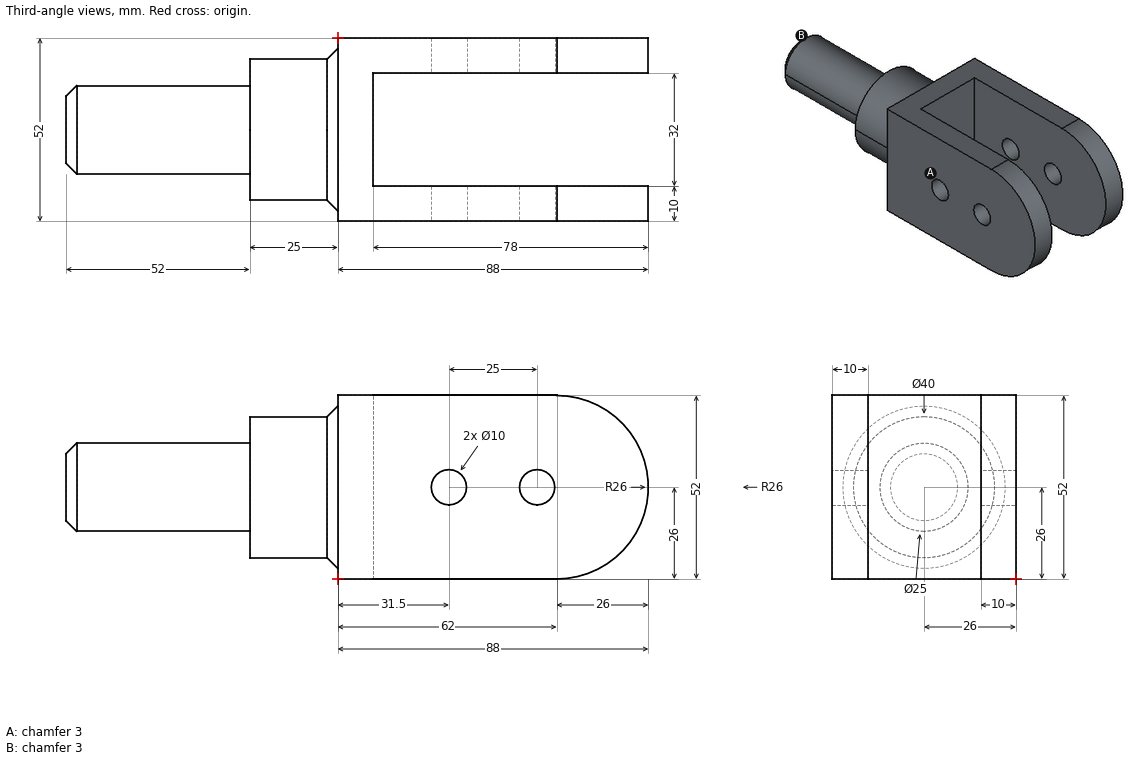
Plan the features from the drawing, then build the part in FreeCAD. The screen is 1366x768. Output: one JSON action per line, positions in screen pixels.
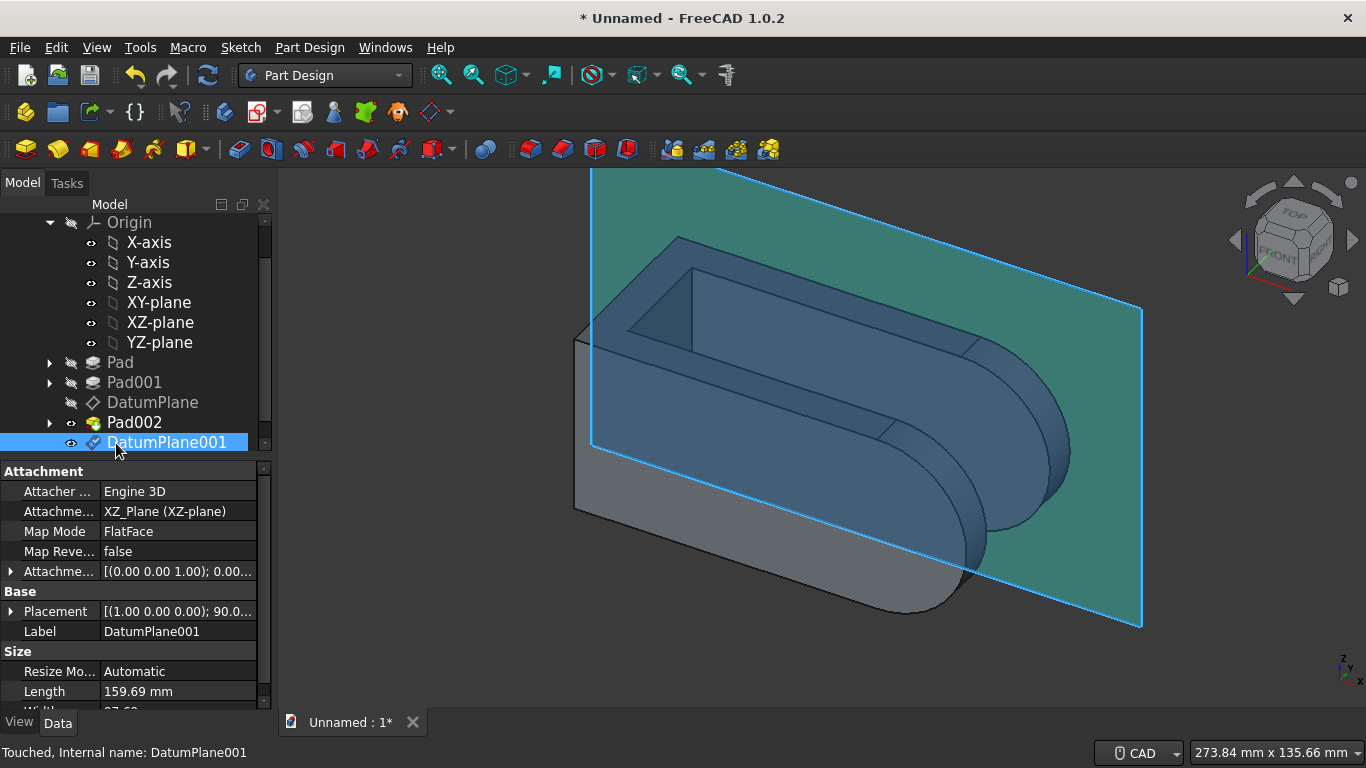
{"action": "left_click", "coordinate": [258, 112]}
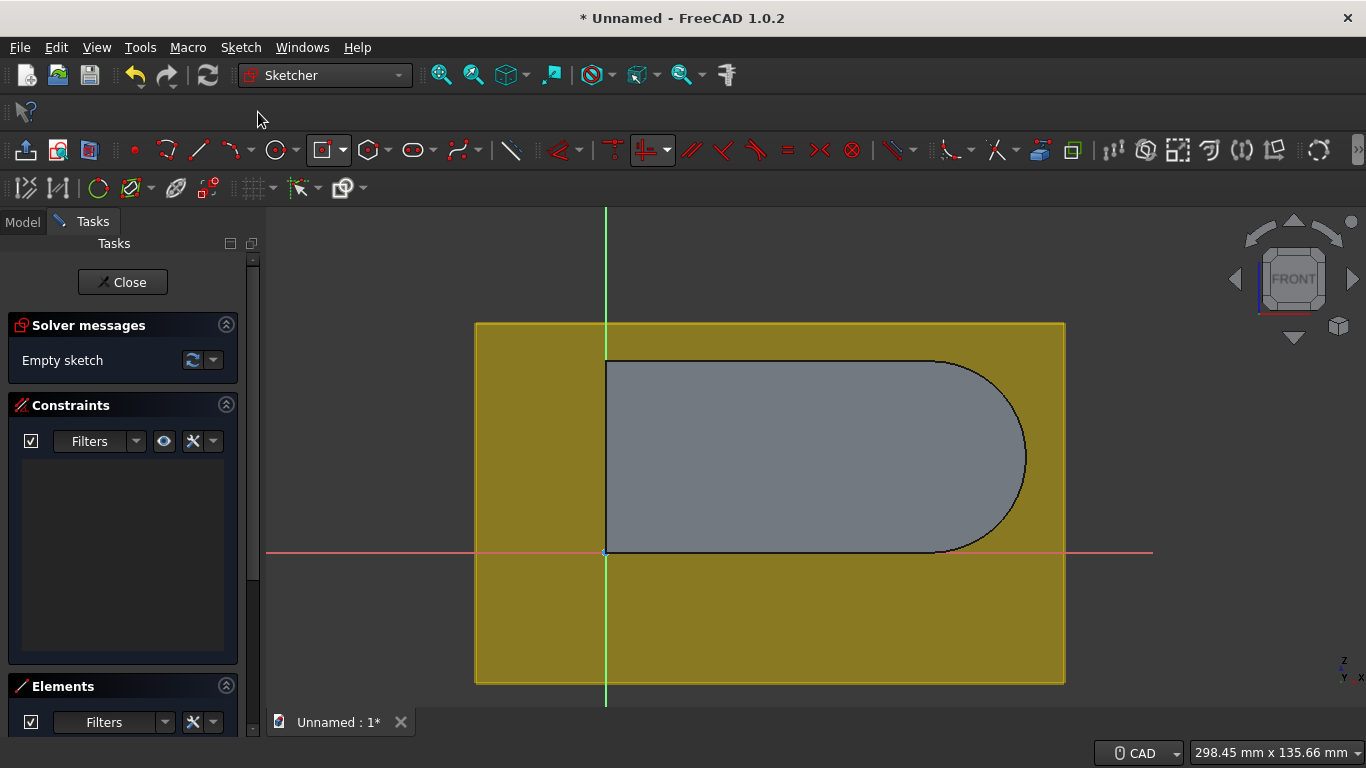
{"action": "left_click", "coordinate": [90, 150]}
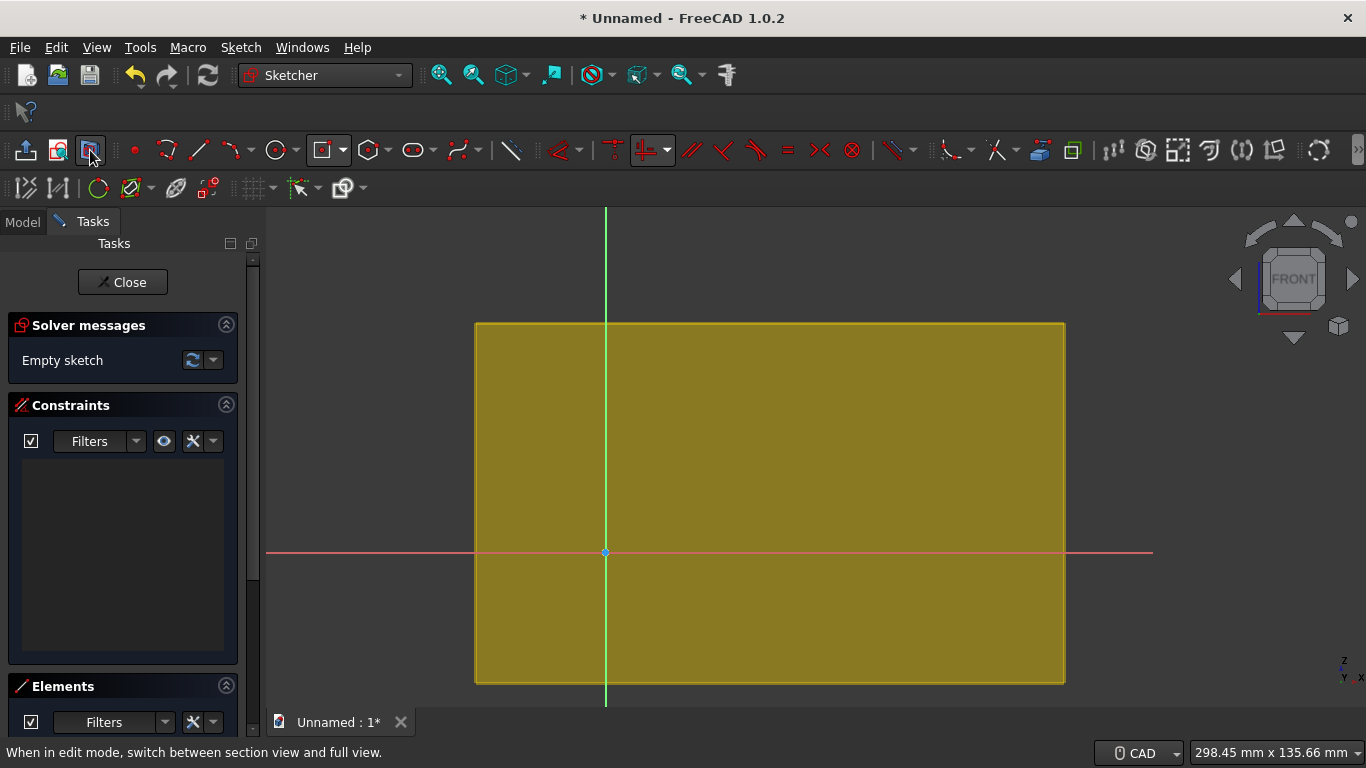
{"action": "scroll", "coordinate": [955, 457], "scroll_direction": "up", "scroll_amount": 2}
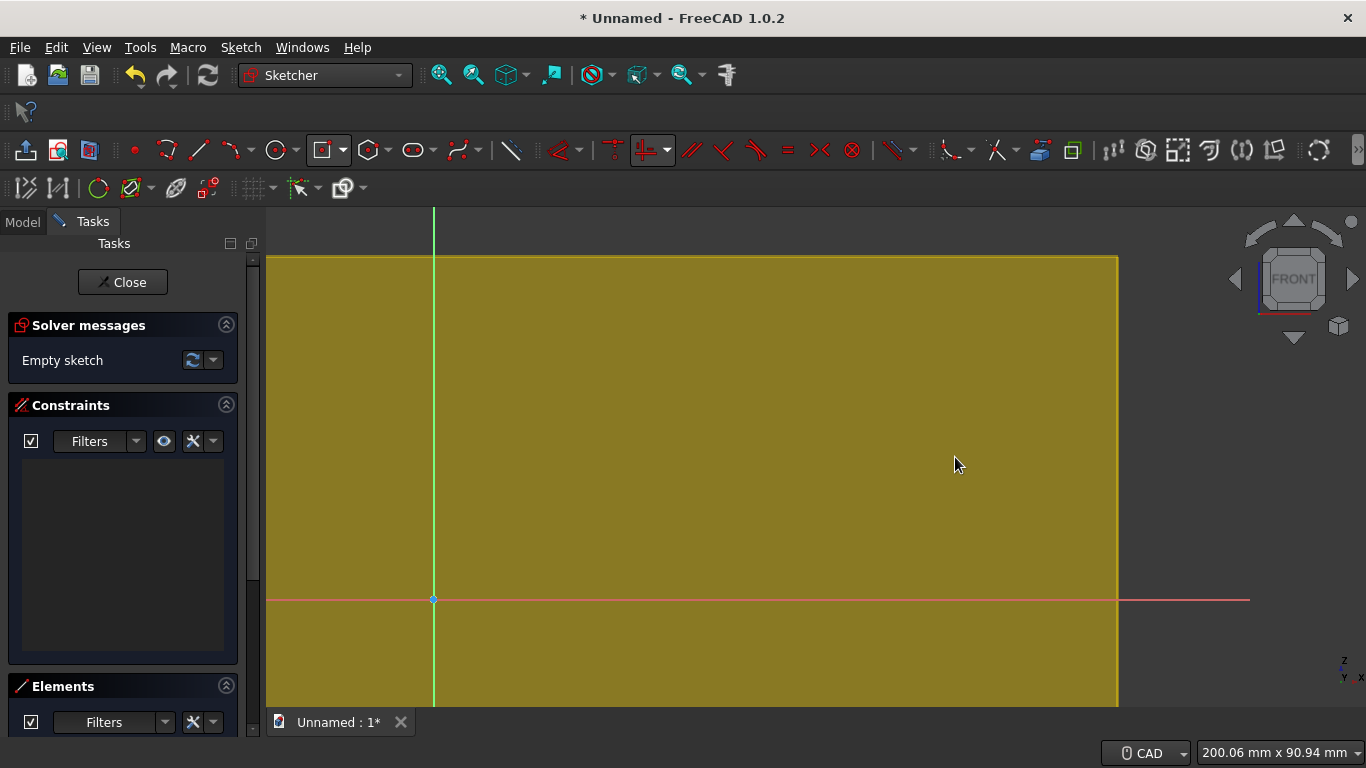
{"action": "left_click", "coordinate": [200, 150]}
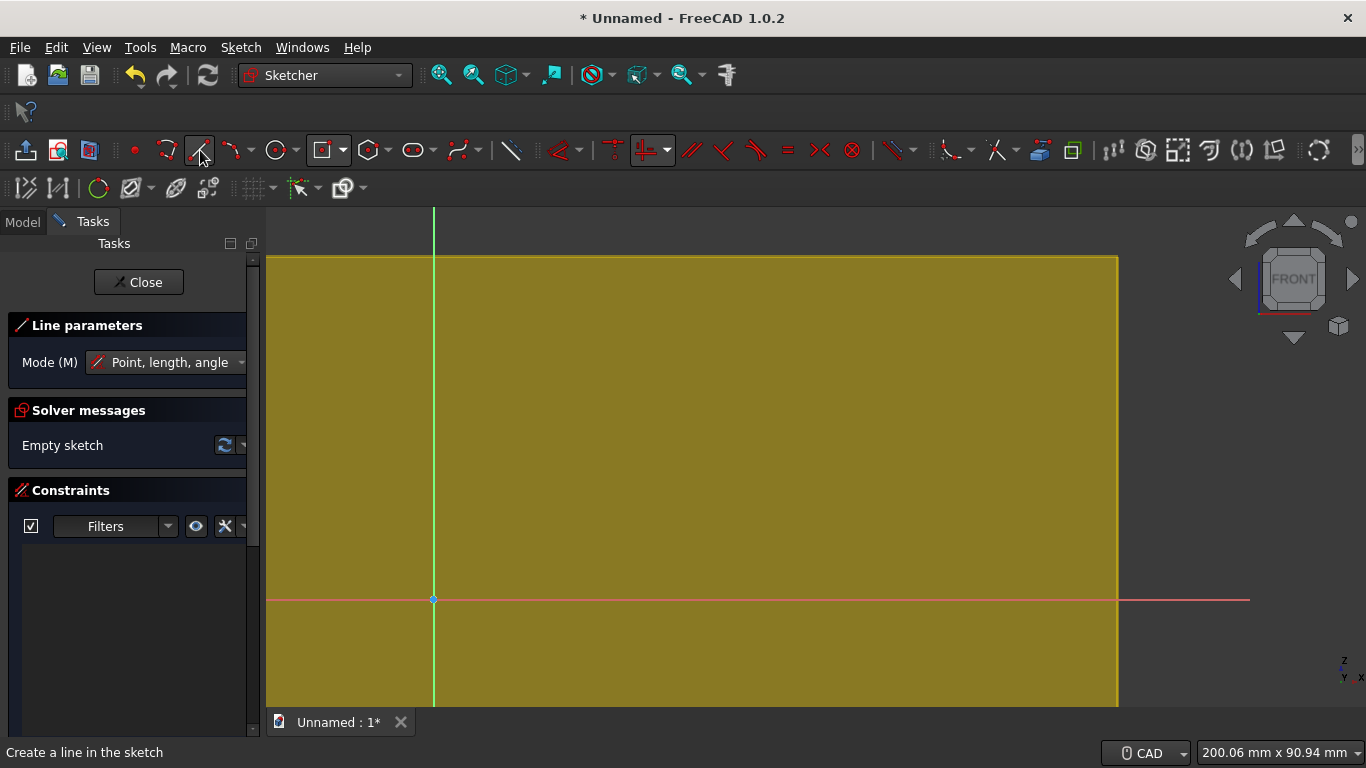
{"action": "left_click", "coordinate": [918, 314]}
{"action": "left_click", "coordinate": [918, 600]}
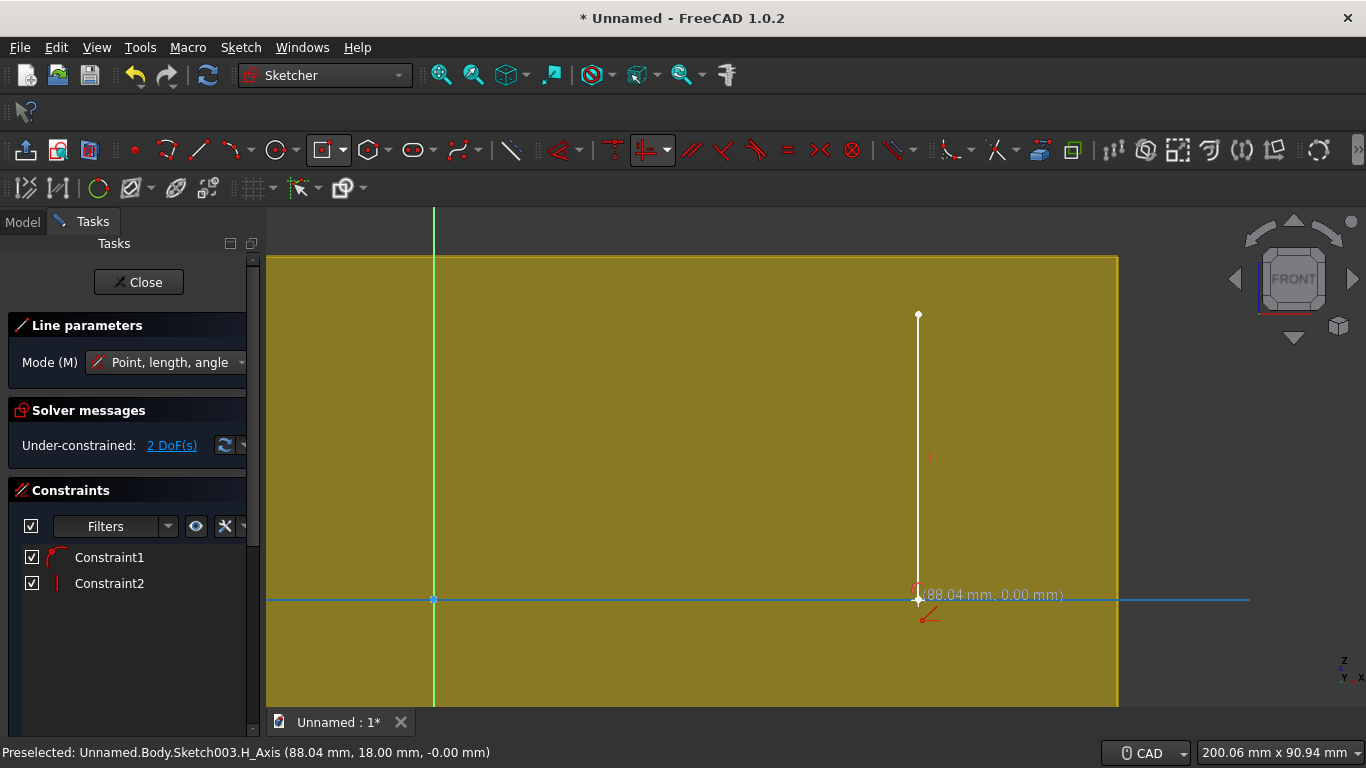
{"action": "left_click", "coordinate": [232, 150]}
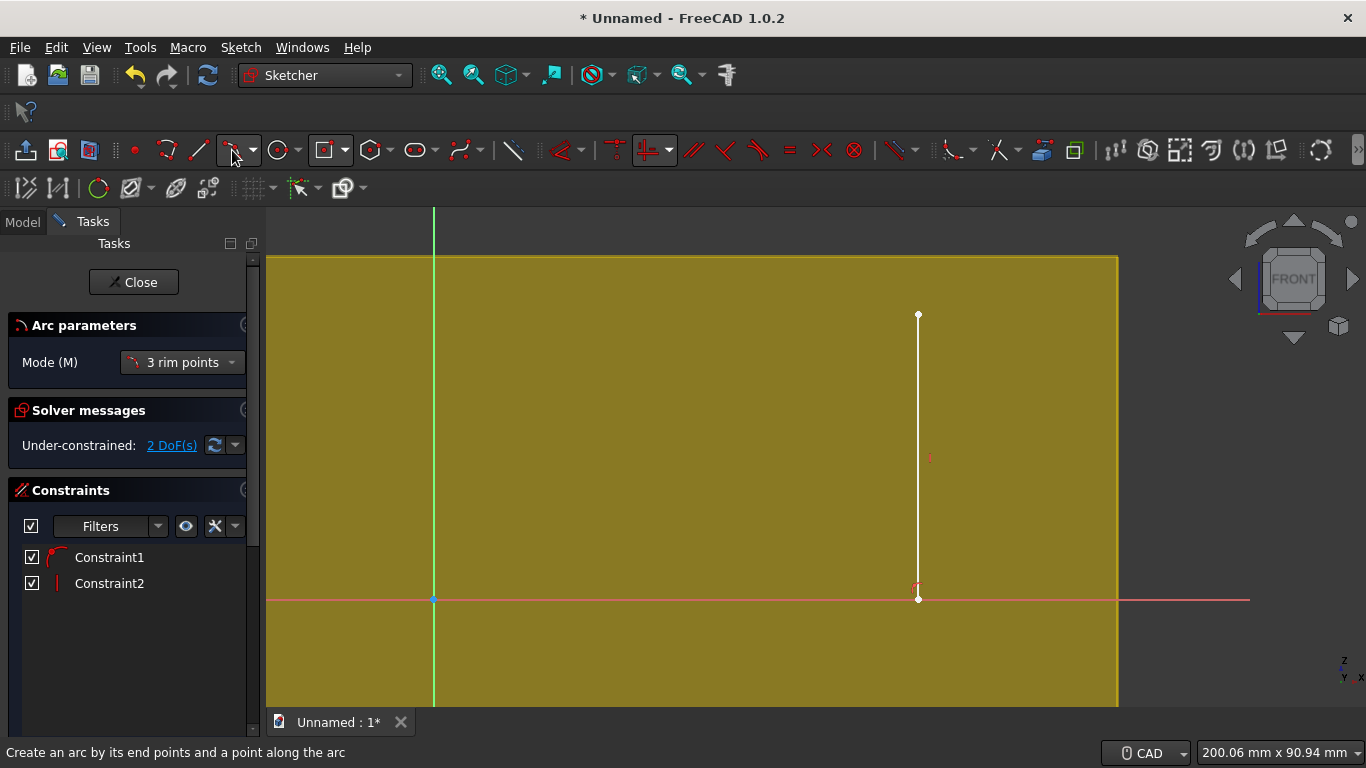
{"action": "left_click", "coordinate": [918, 600]}
{"action": "left_click", "coordinate": [918, 315]}
{"action": "left_click", "coordinate": [1061, 457]}
{"action": "key", "text": "Escape"}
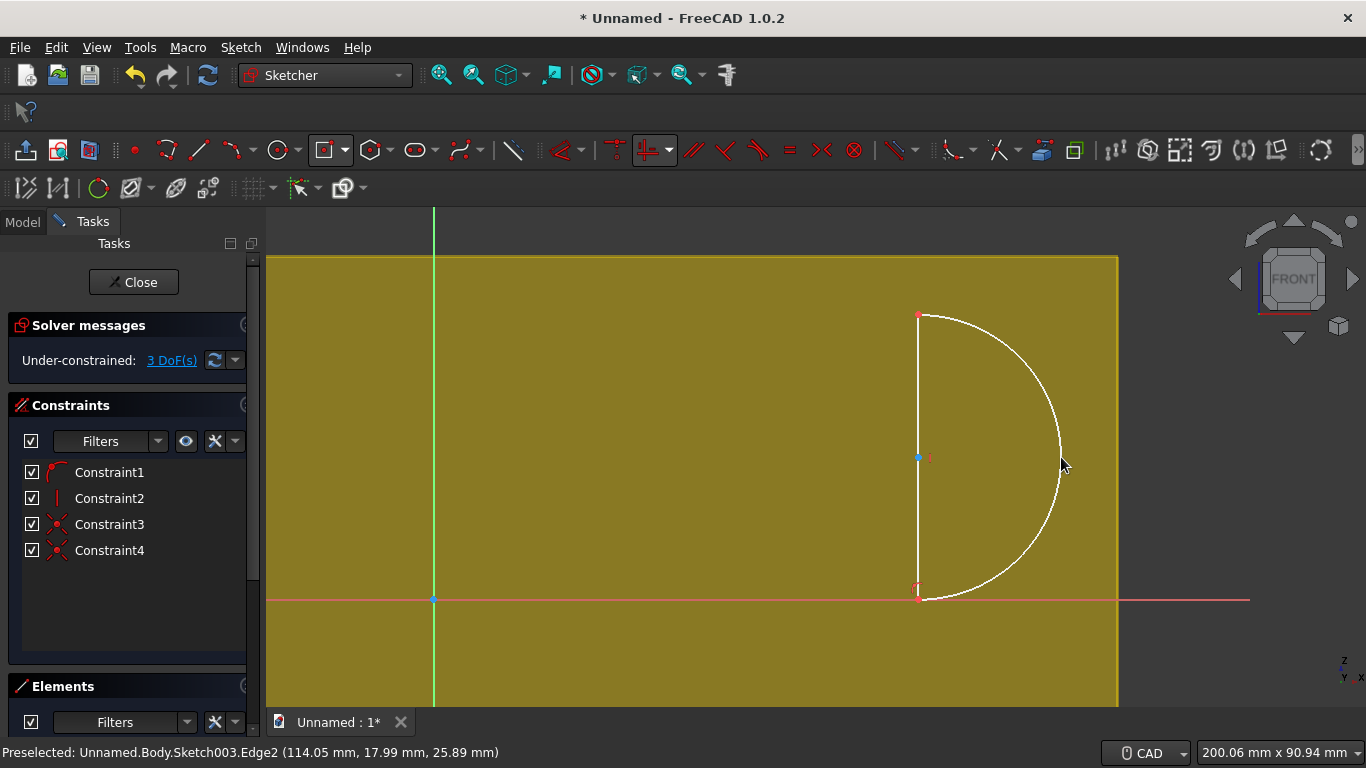
{"action": "left_click", "coordinate": [560, 150]}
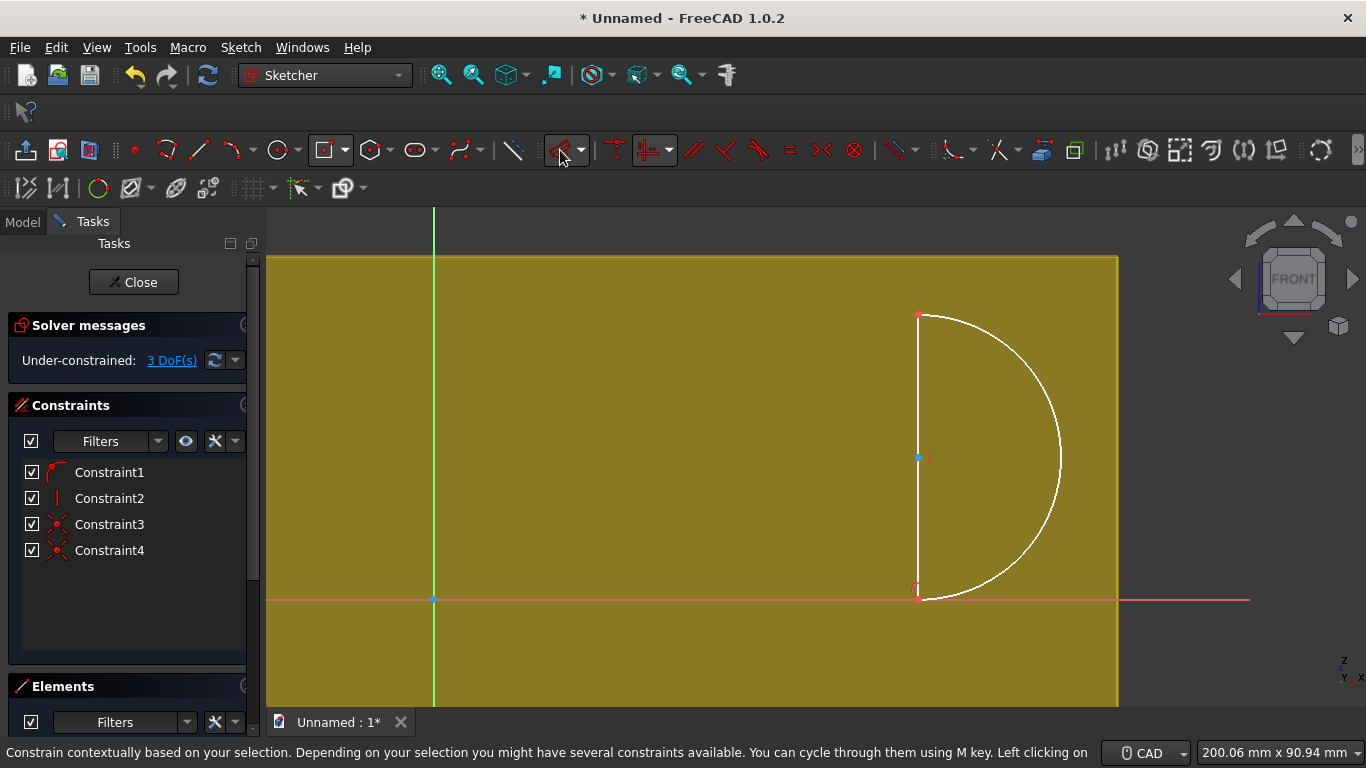
{"action": "left_click", "coordinate": [1034, 541]}
{"action": "left_click", "coordinate": [1060, 560]}